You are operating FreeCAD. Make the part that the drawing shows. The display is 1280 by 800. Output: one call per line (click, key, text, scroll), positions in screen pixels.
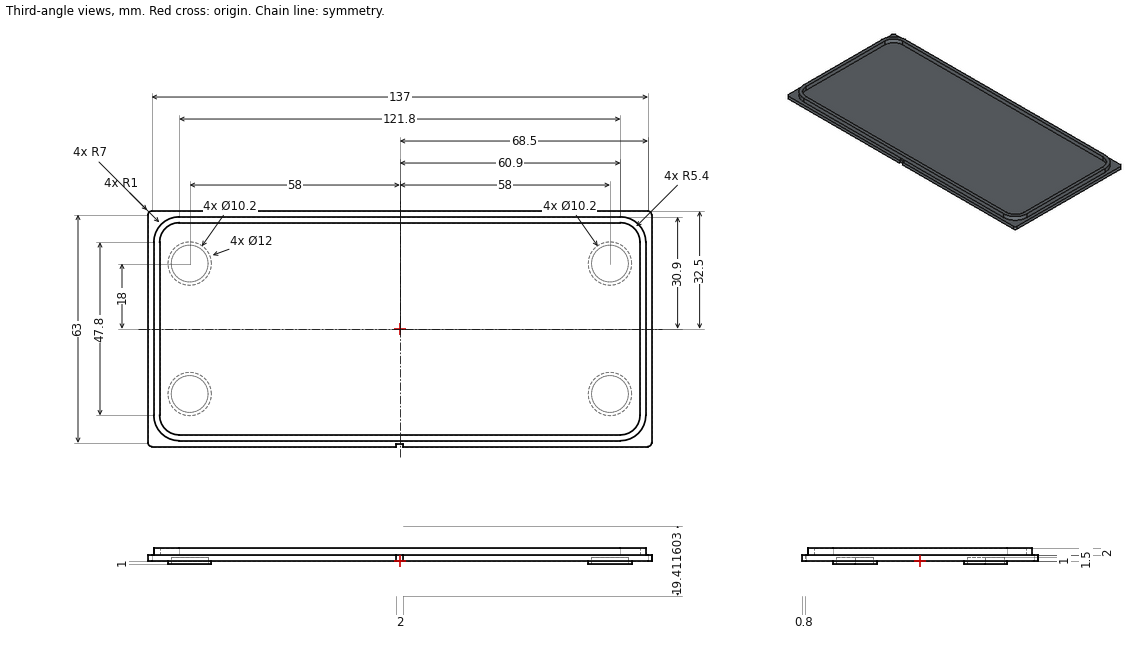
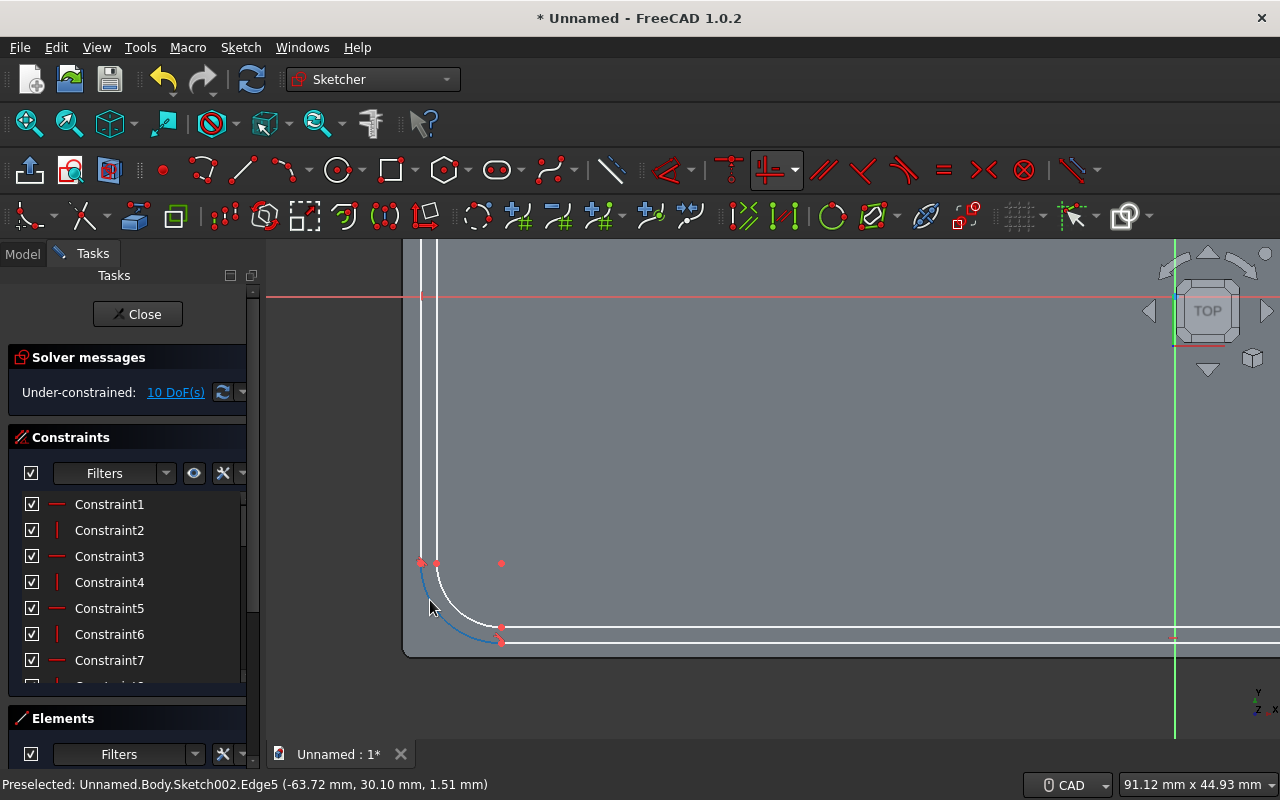
click(430, 599)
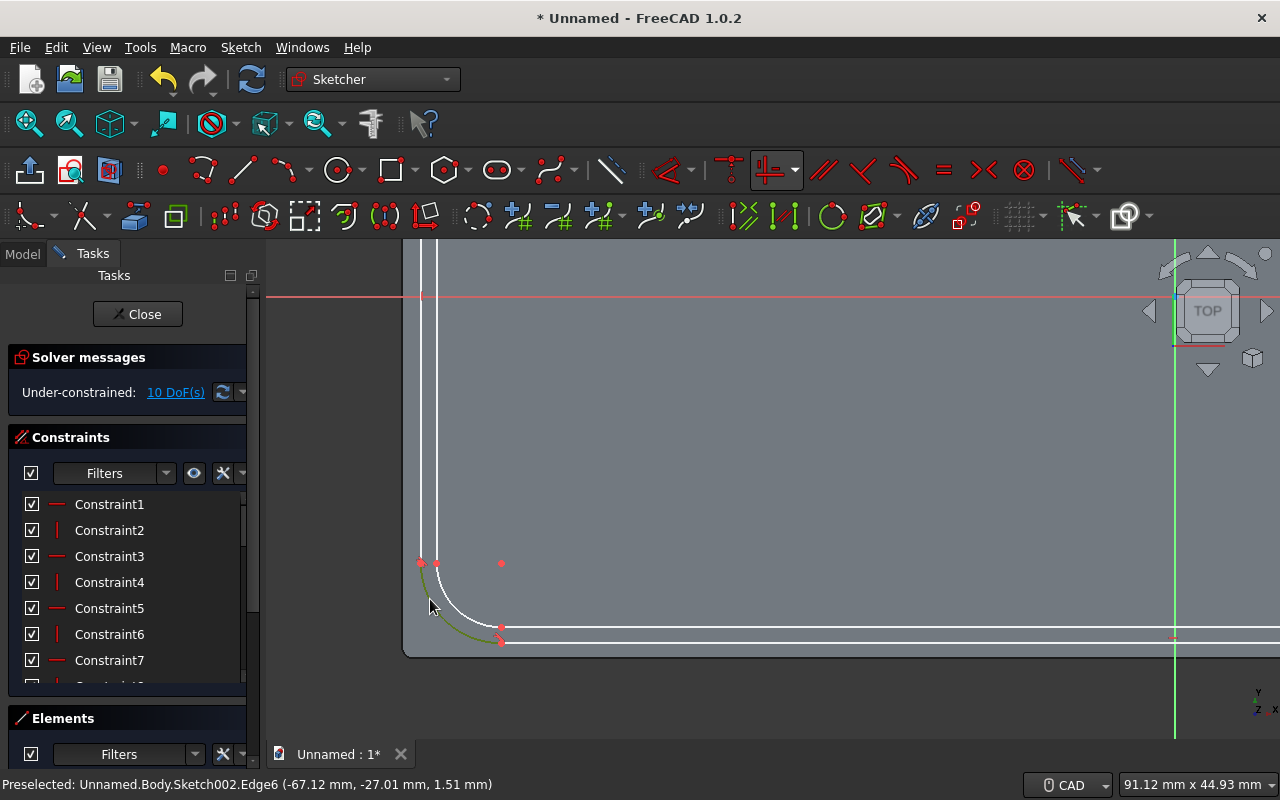
scroll(430, 601, down, 5)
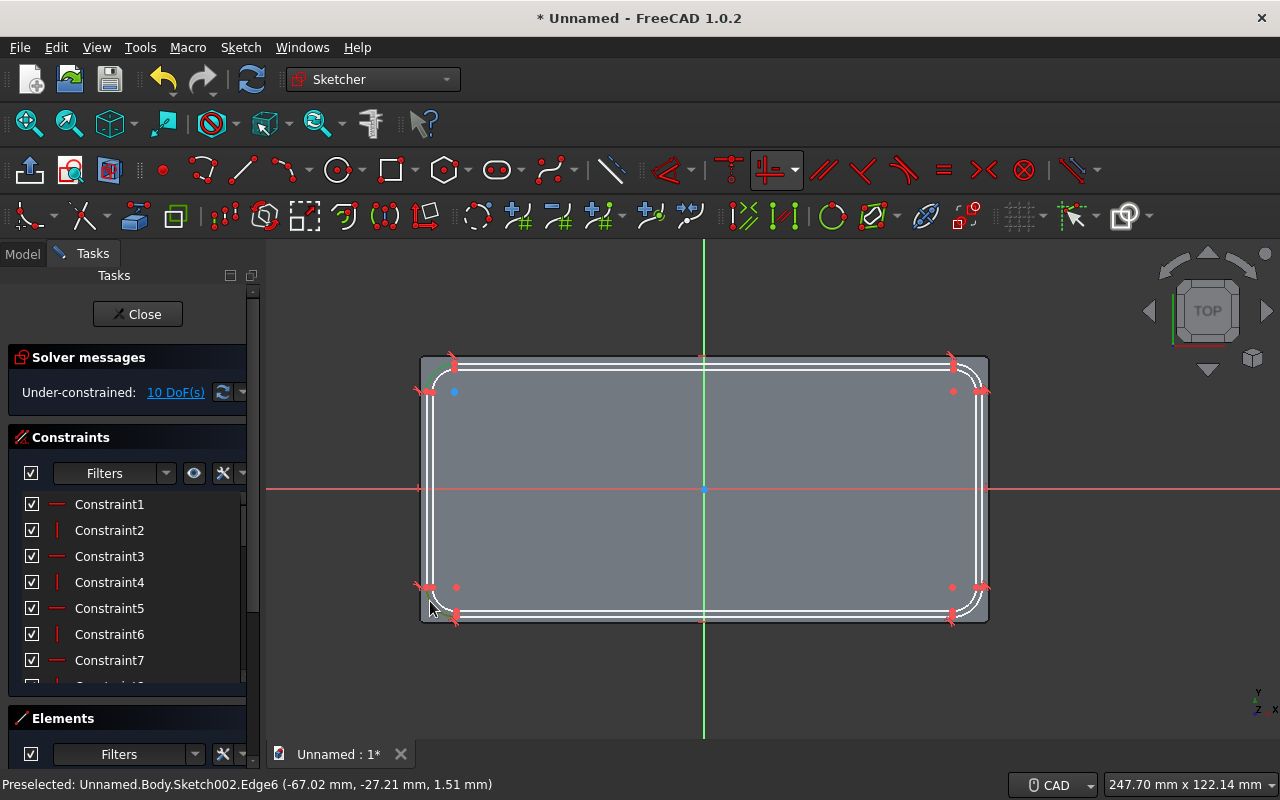
scroll(966, 614, up, 5)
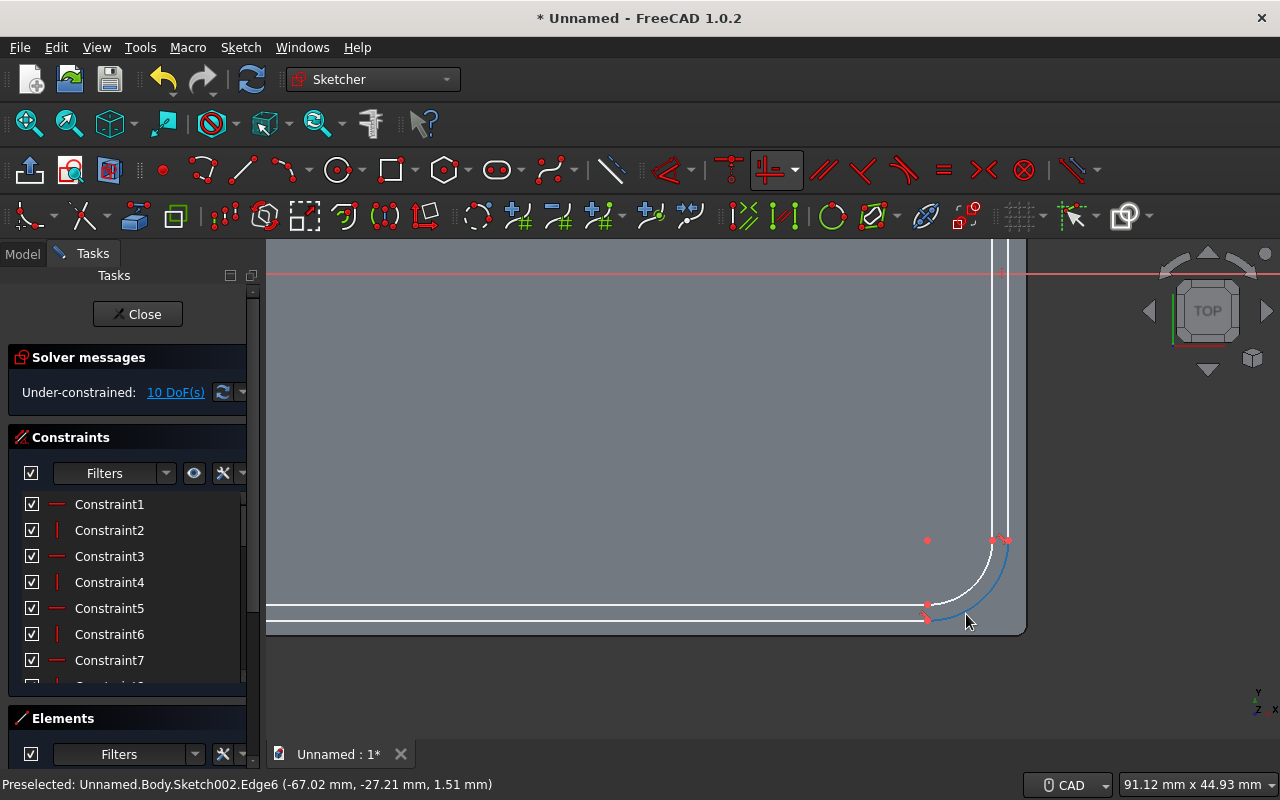
click(964, 612)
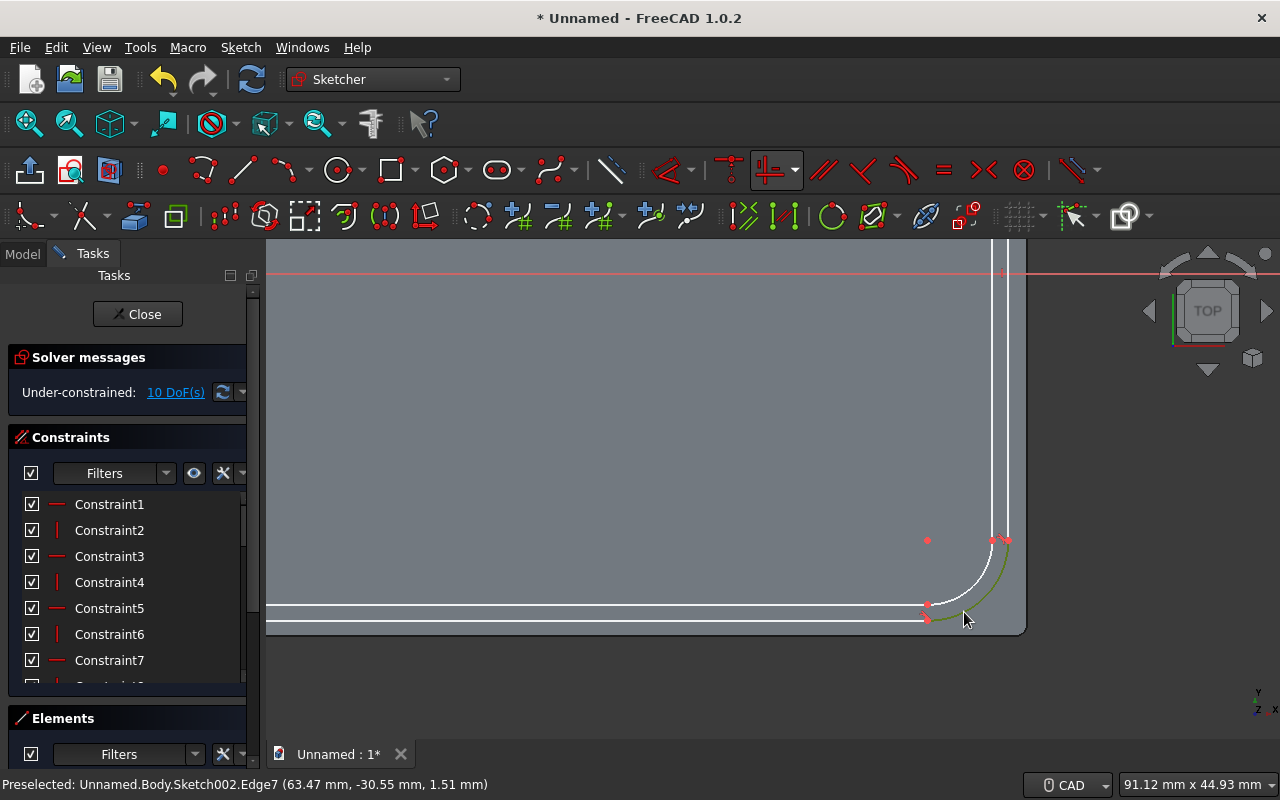
scroll(967, 614, down, 5)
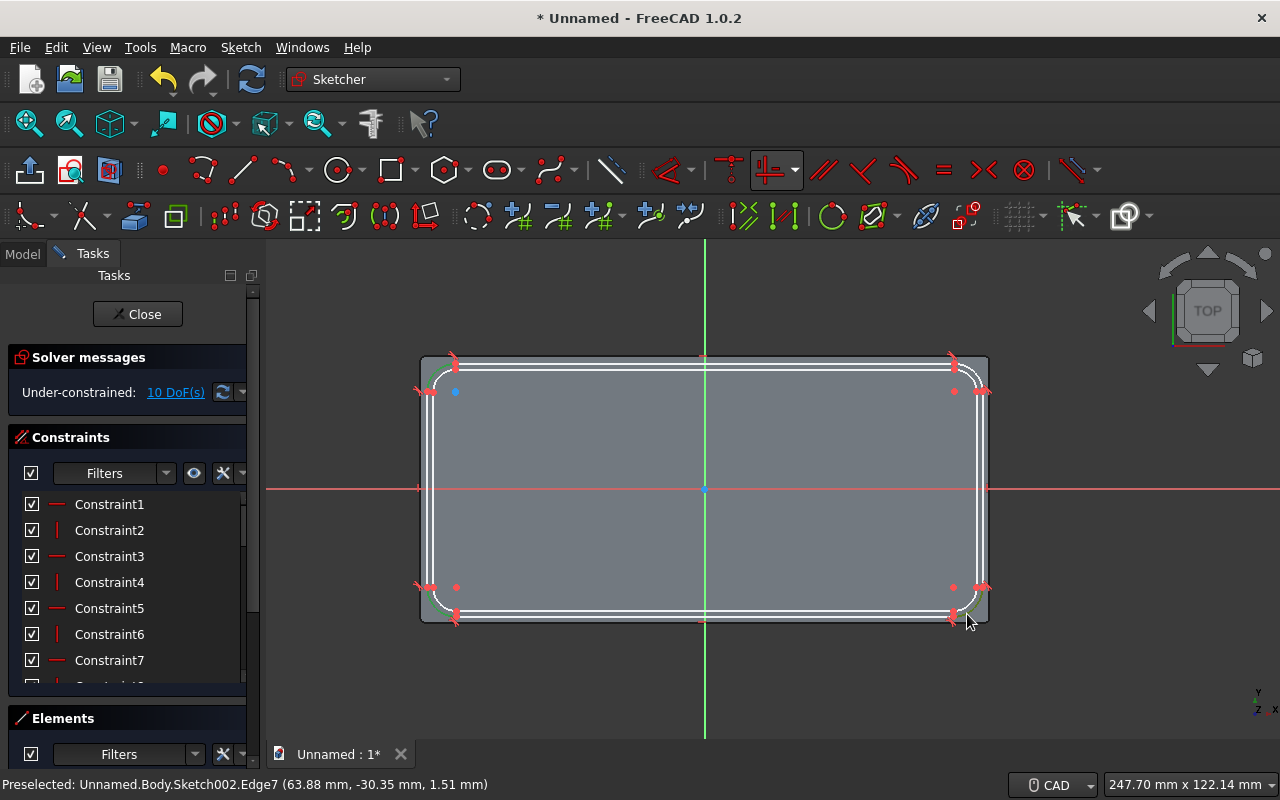
scroll(980, 379, up, 5)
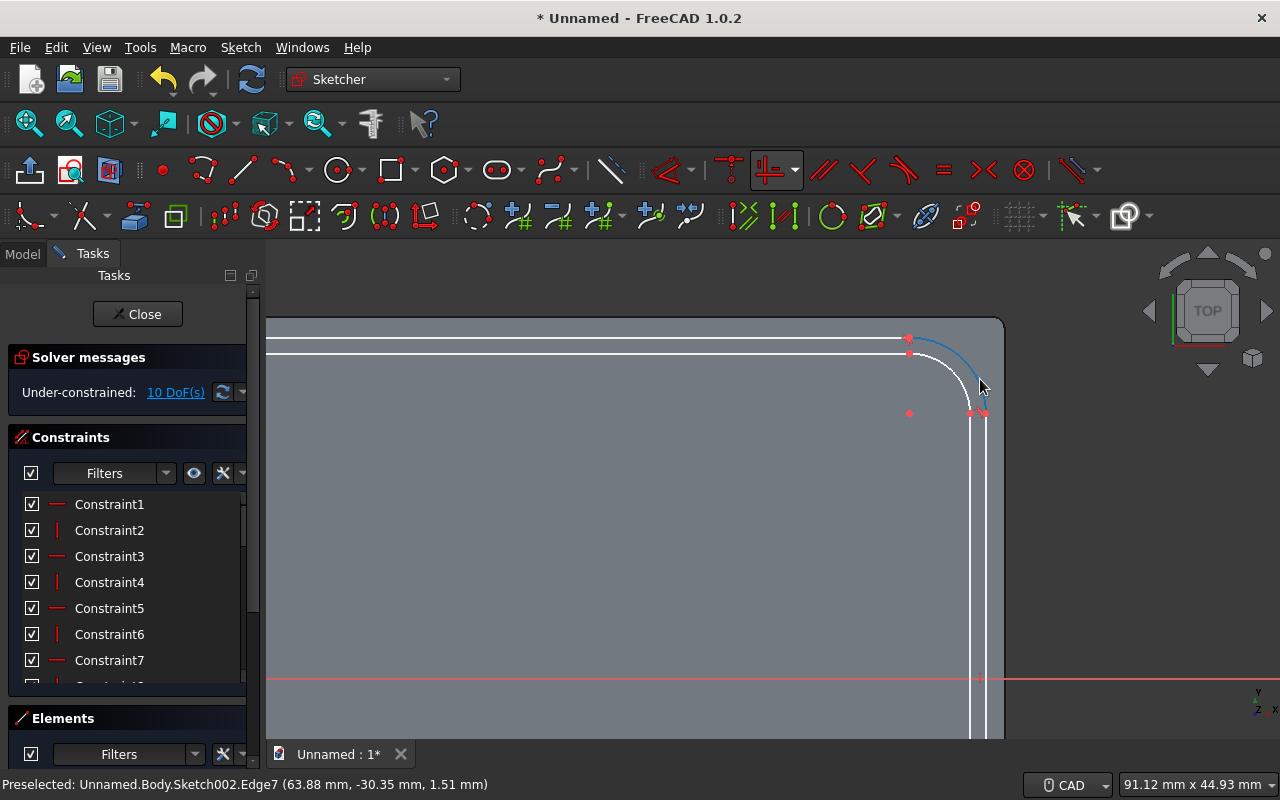
click(978, 379)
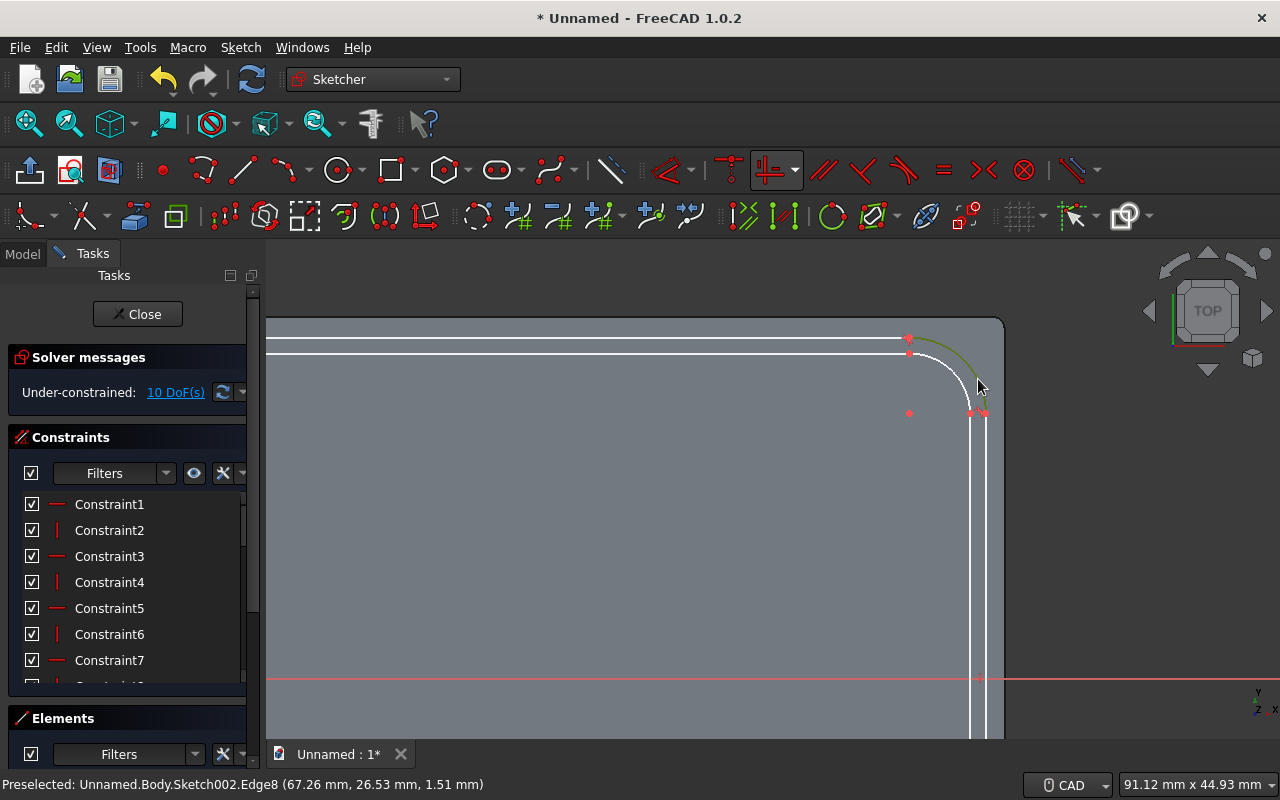
click(944, 170)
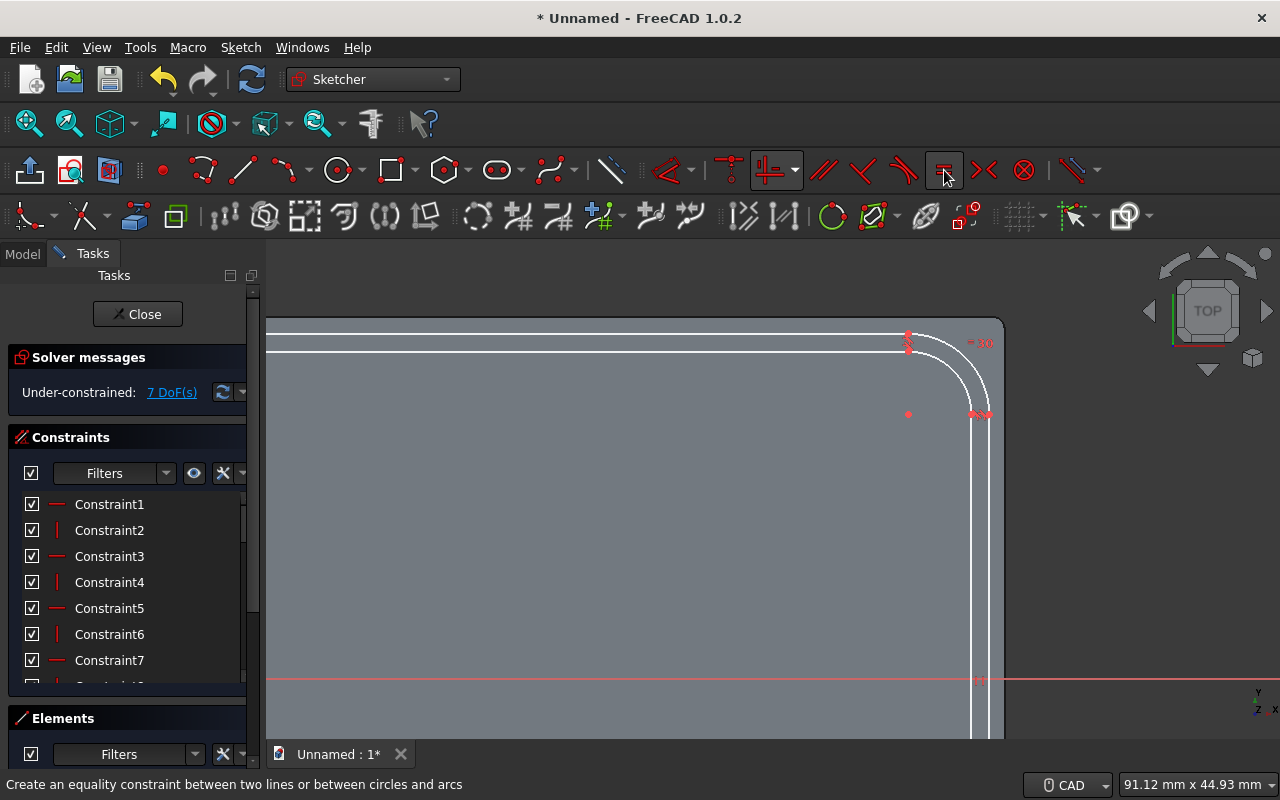
click(965, 386)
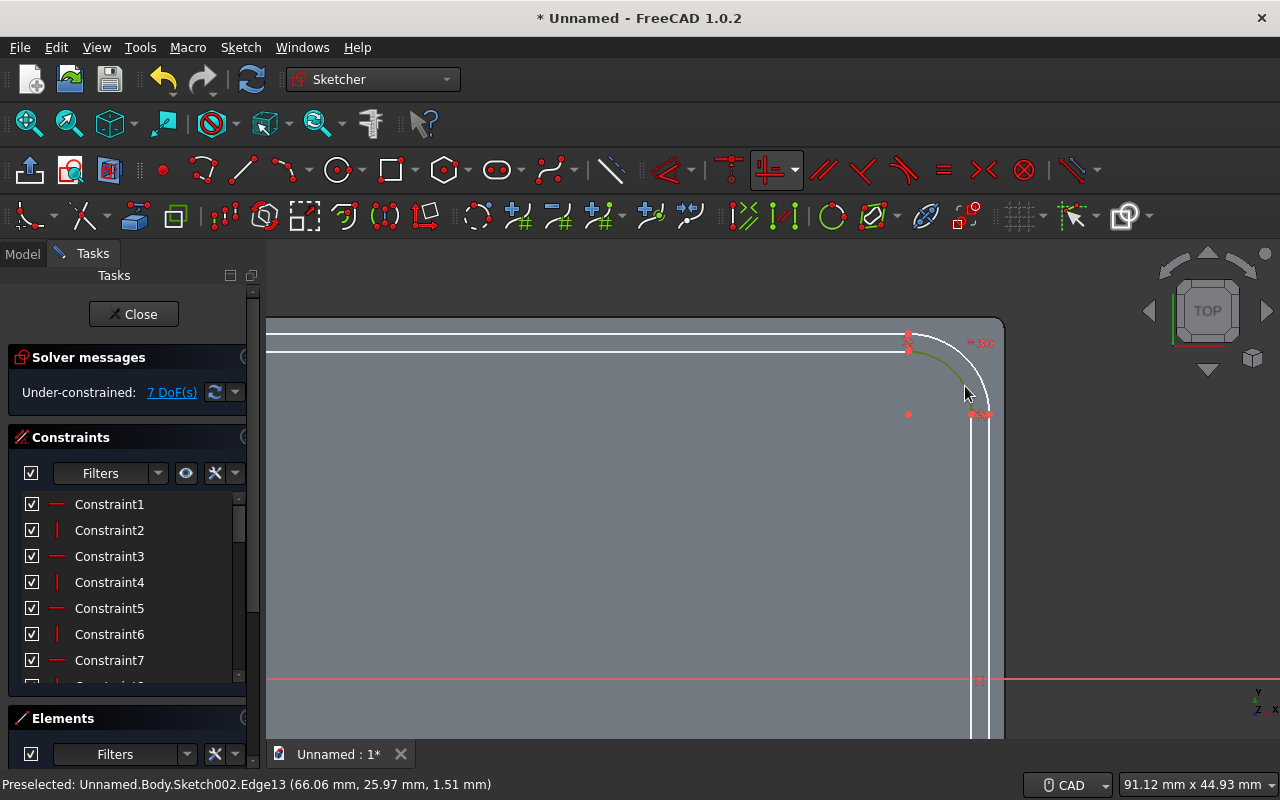
scroll(980, 379, down, 5)